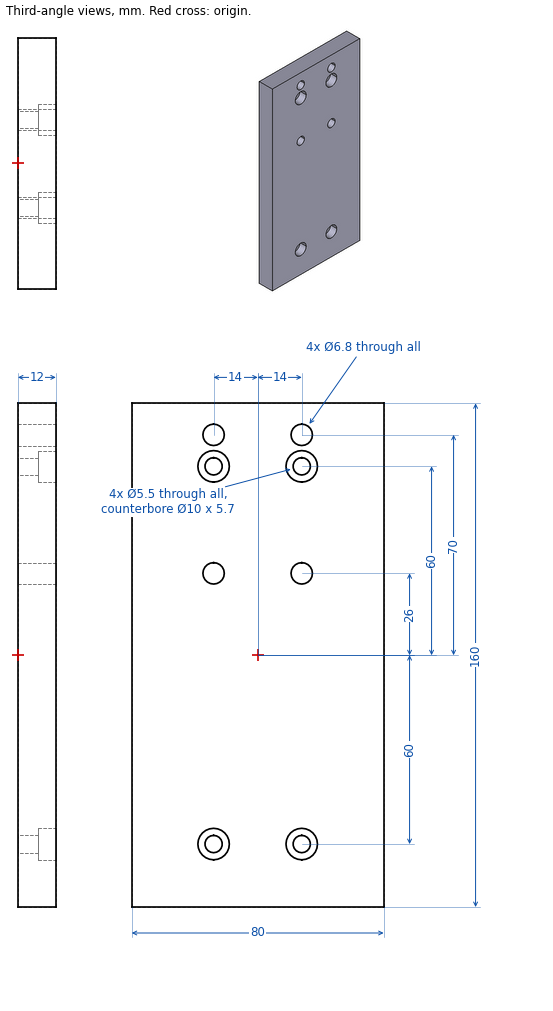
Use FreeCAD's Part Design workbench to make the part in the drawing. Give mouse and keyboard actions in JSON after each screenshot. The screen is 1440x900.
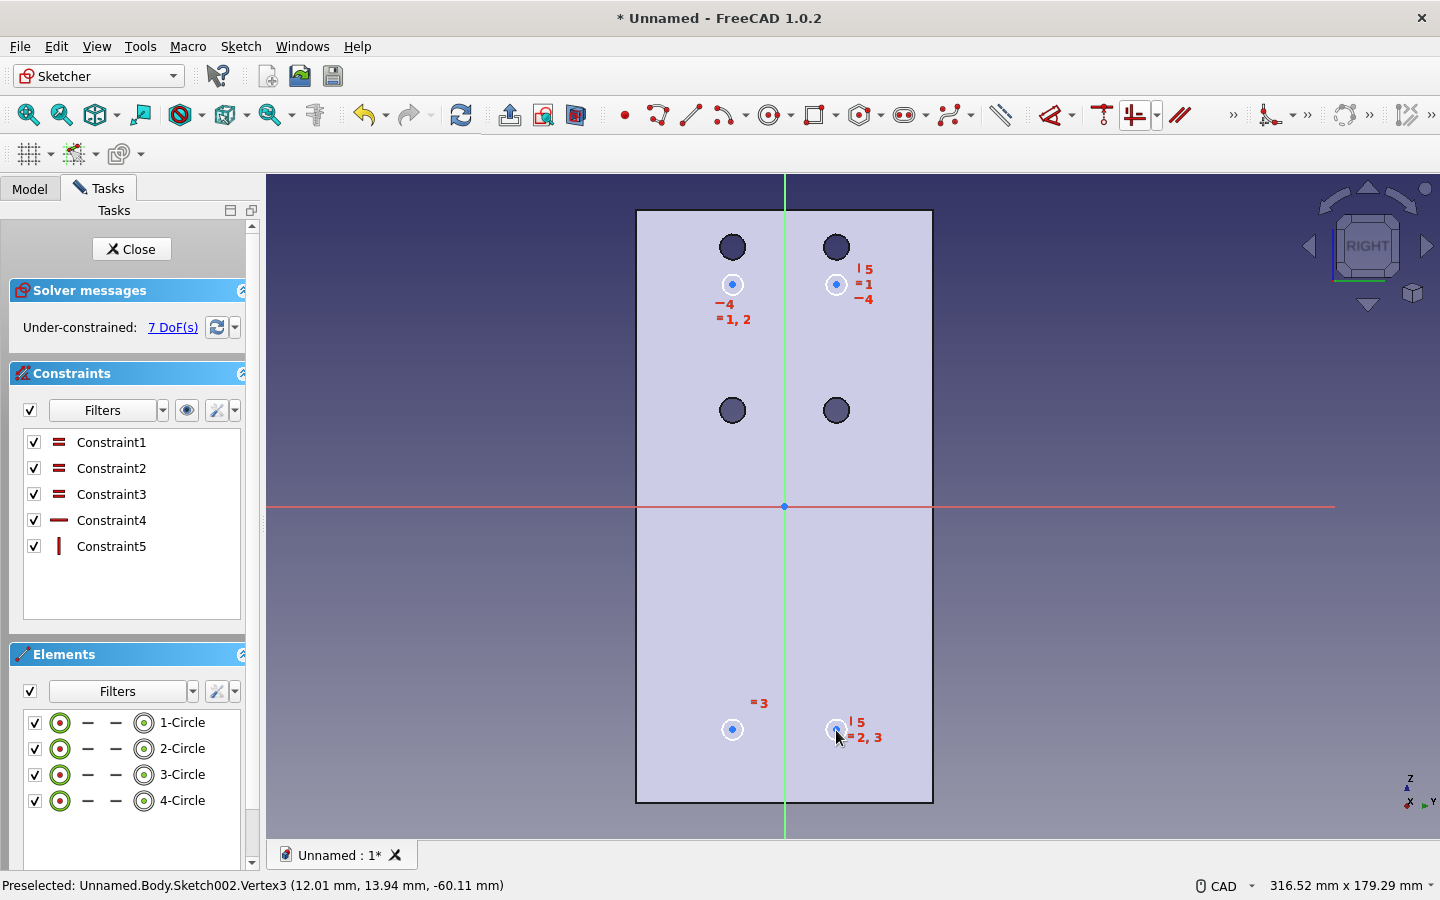
{"action": "left_click", "coordinate": [733, 285]}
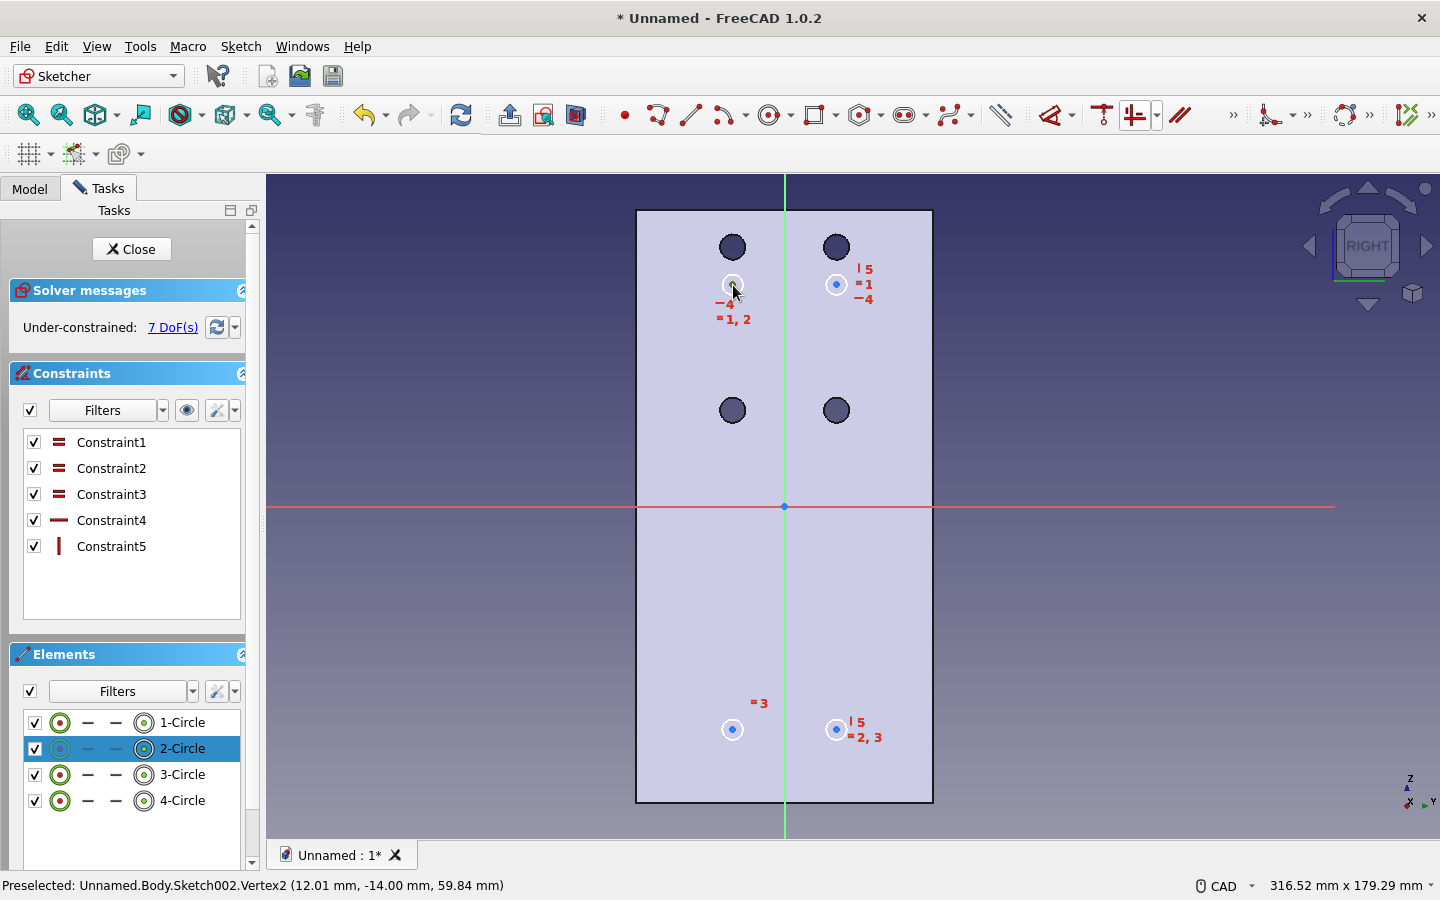
{"action": "left_click", "coordinate": [733, 730]}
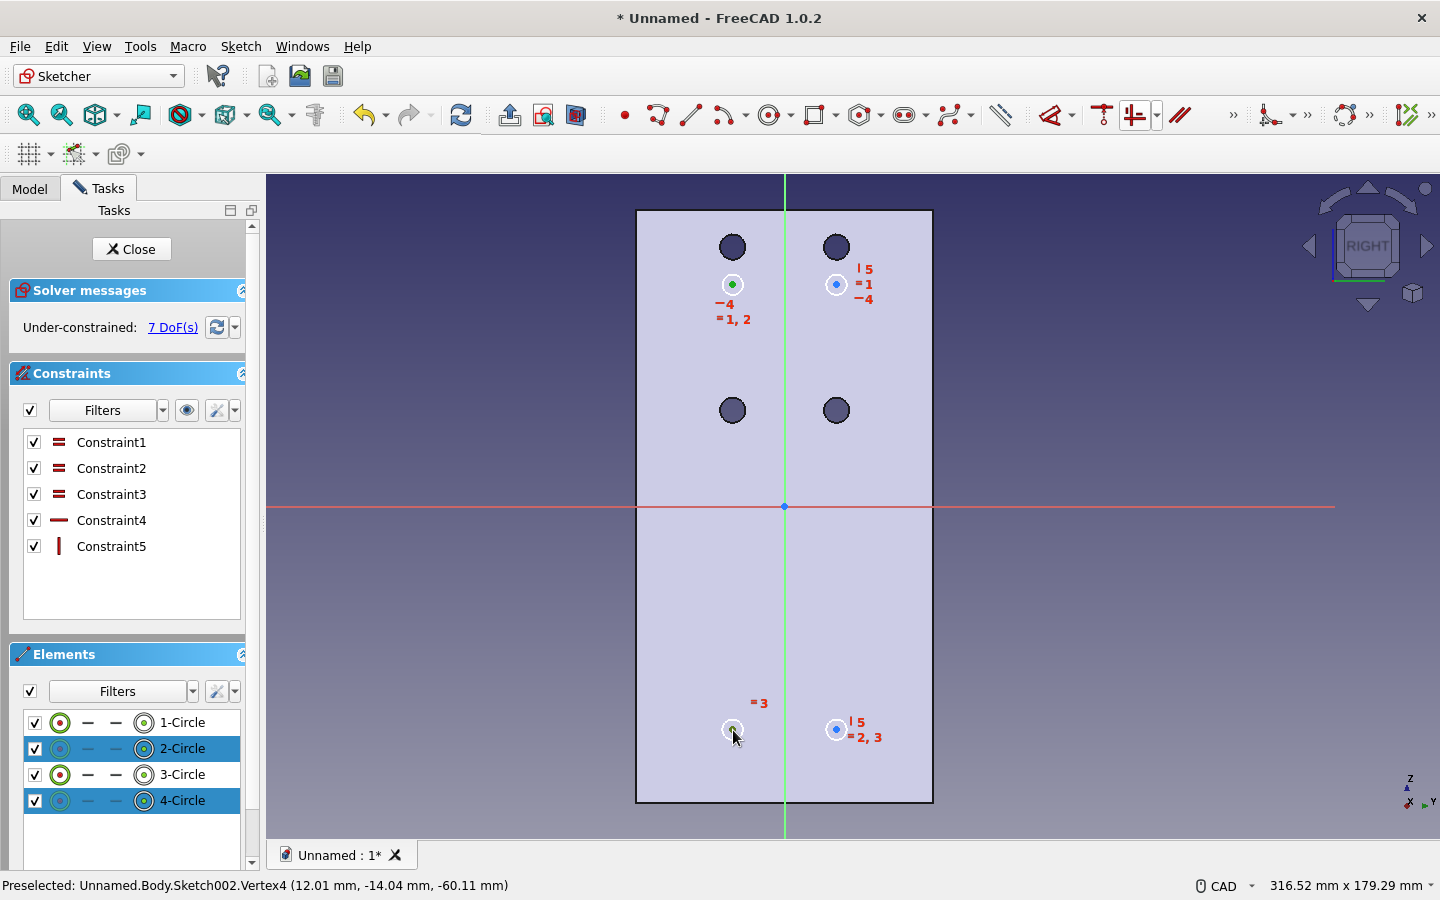
{"action": "left_click", "coordinate": [1156, 116]}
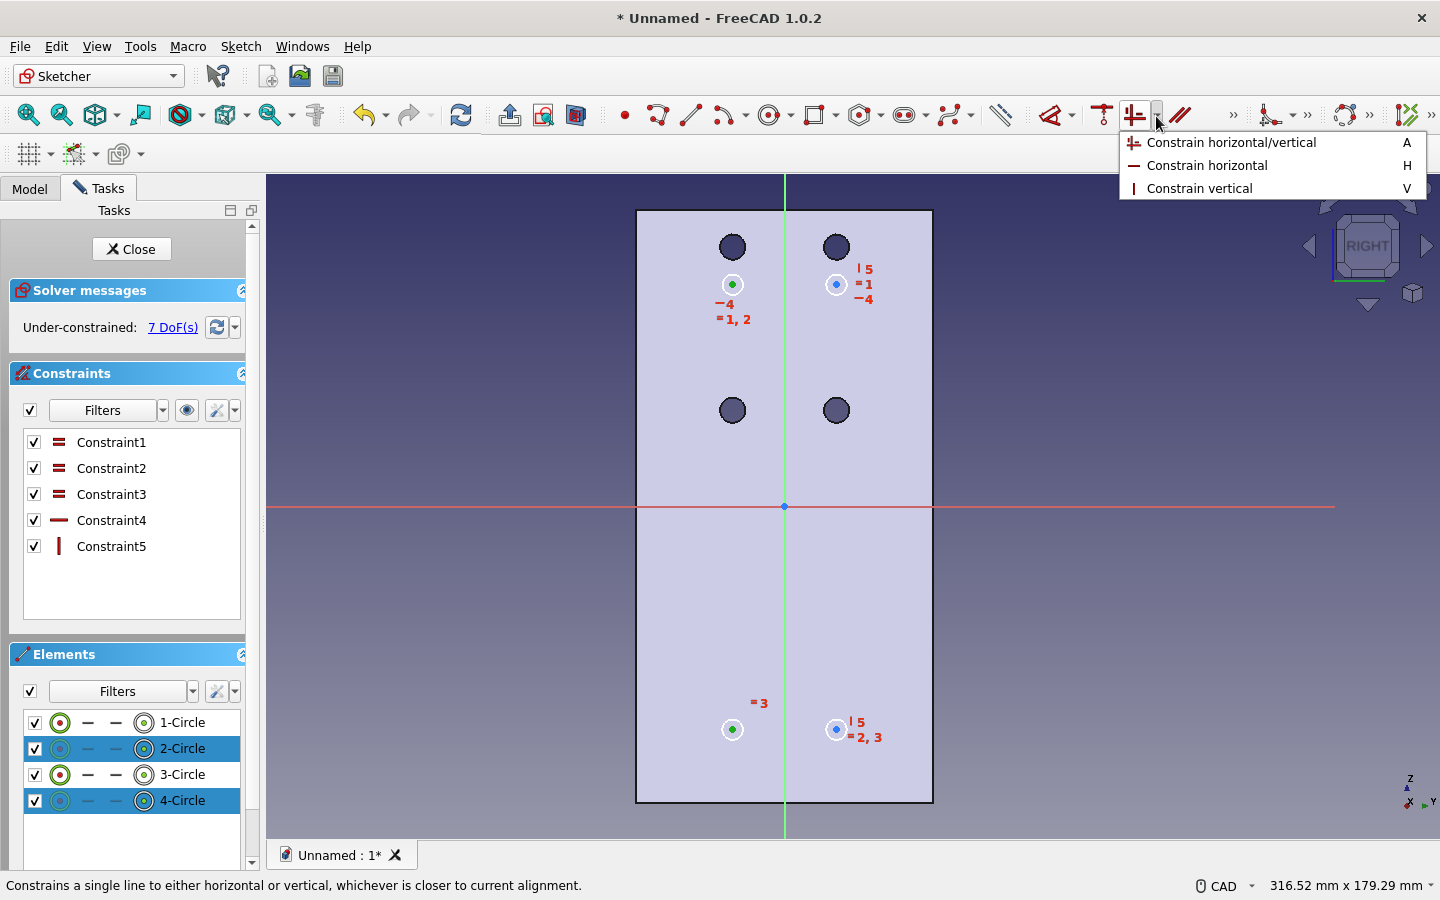
{"action": "left_click", "coordinate": [1273, 188]}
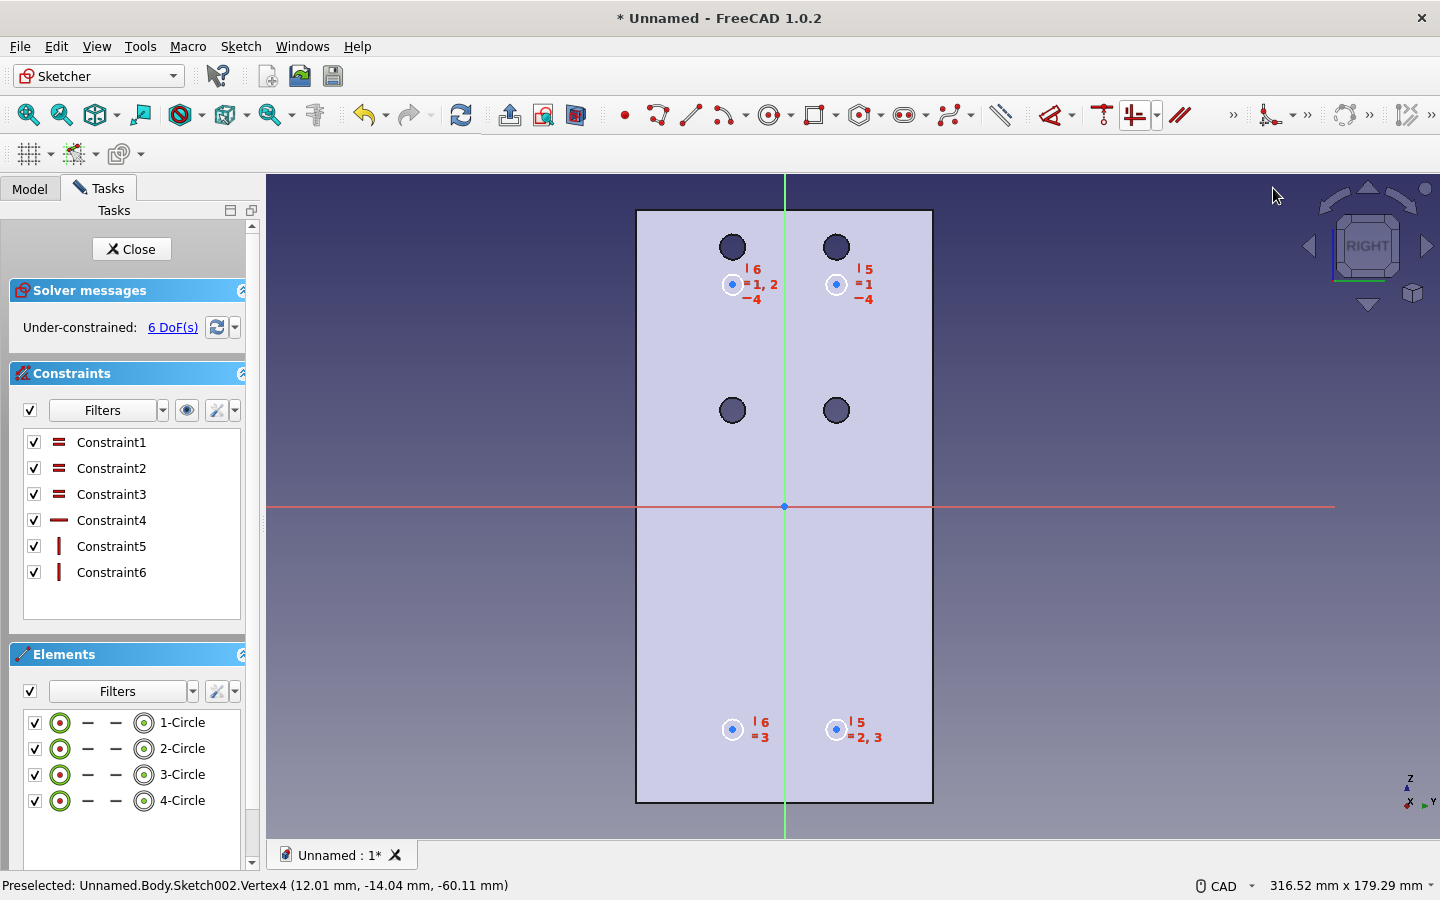
{"action": "left_click", "coordinate": [837, 730]}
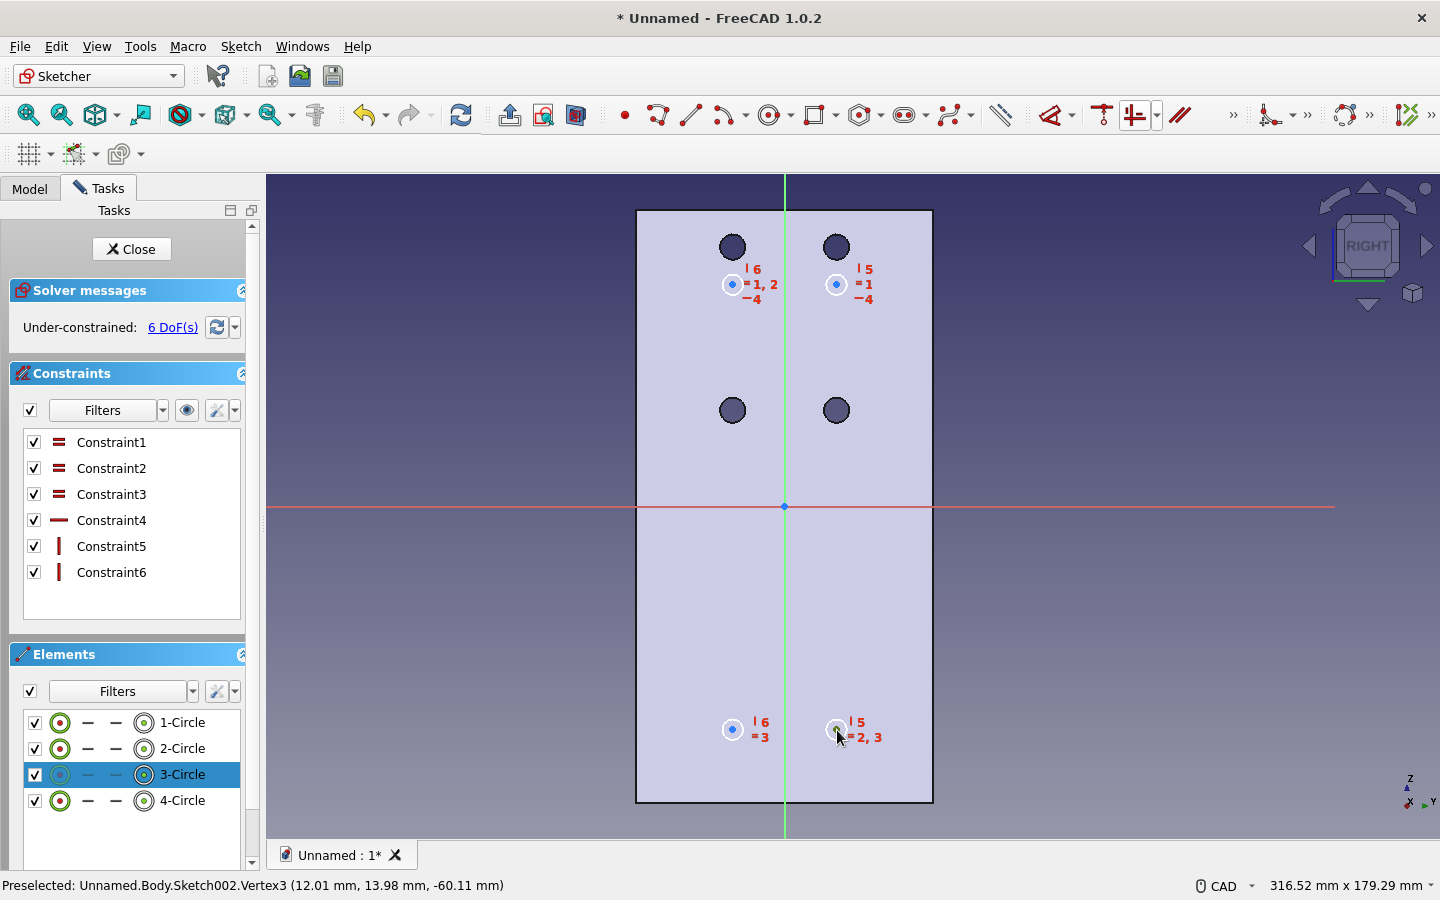
{"action": "left_click", "coordinate": [733, 730]}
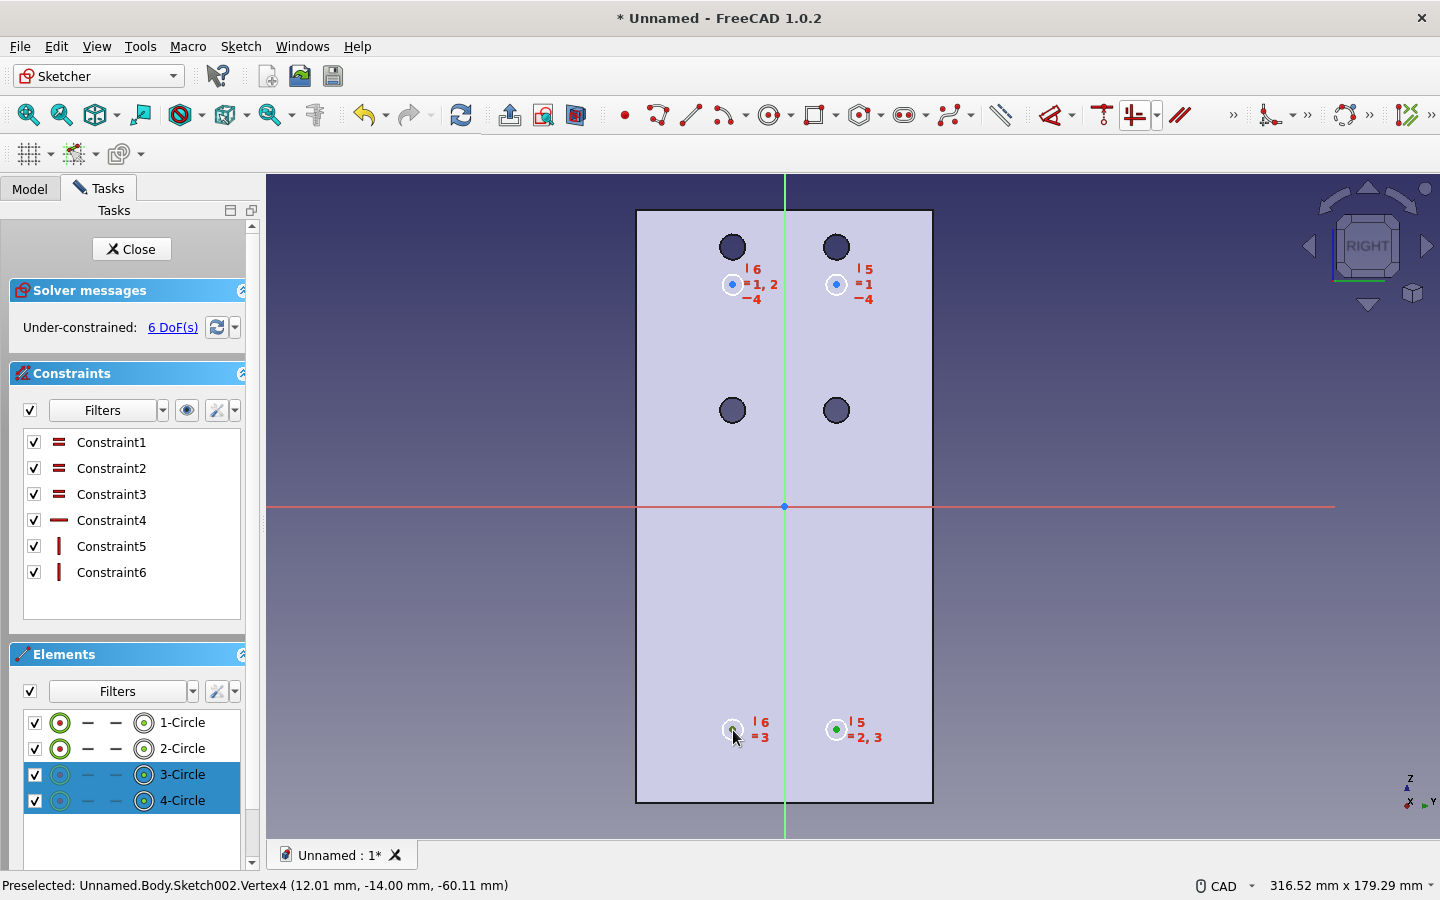
{"action": "left_click", "coordinate": [1156, 116]}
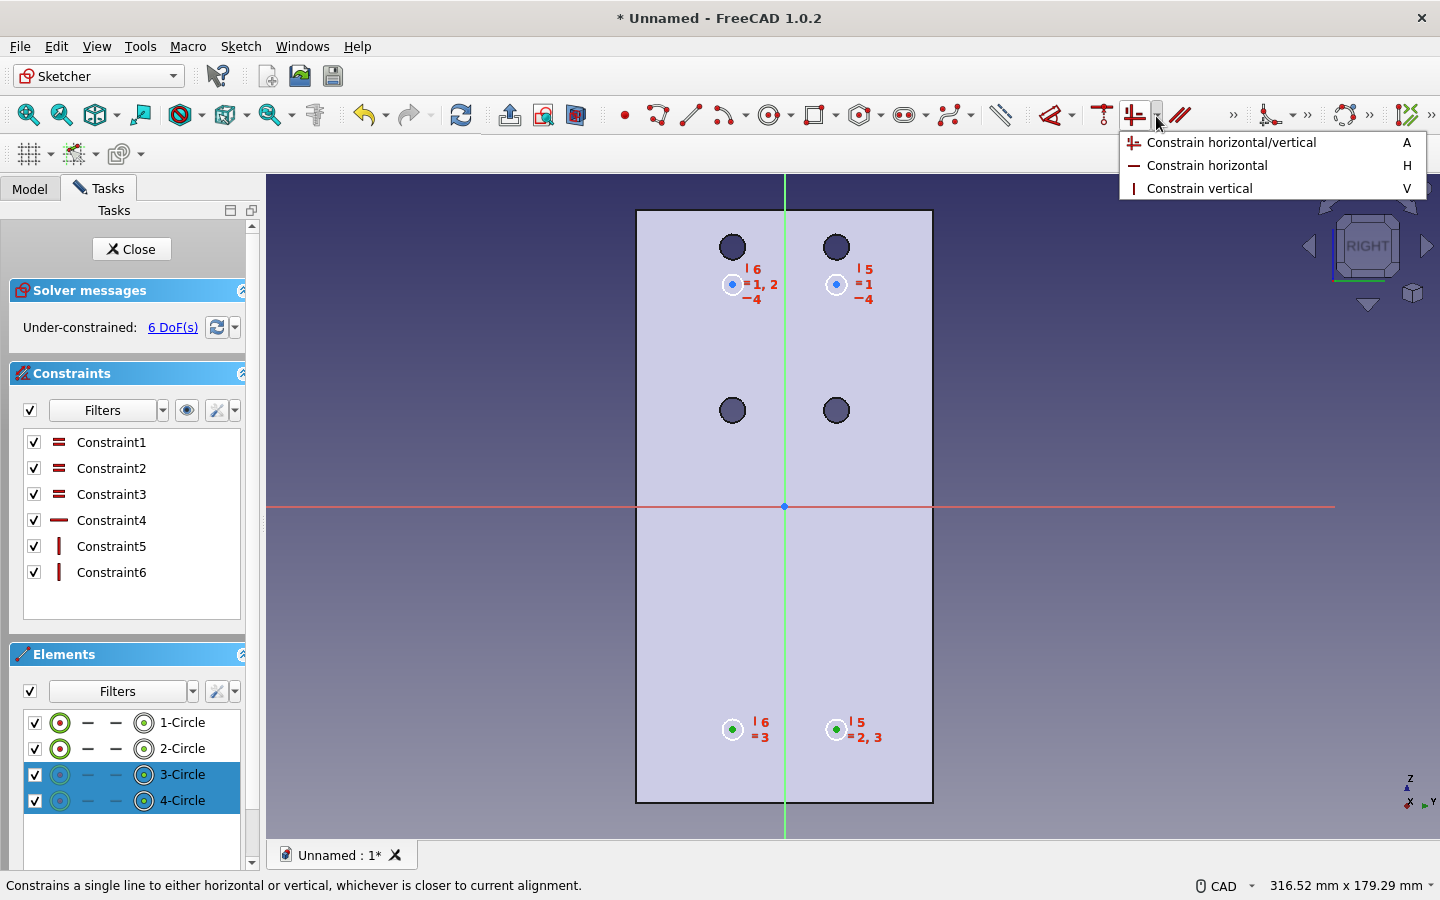
{"action": "left_click", "coordinate": [1273, 166]}